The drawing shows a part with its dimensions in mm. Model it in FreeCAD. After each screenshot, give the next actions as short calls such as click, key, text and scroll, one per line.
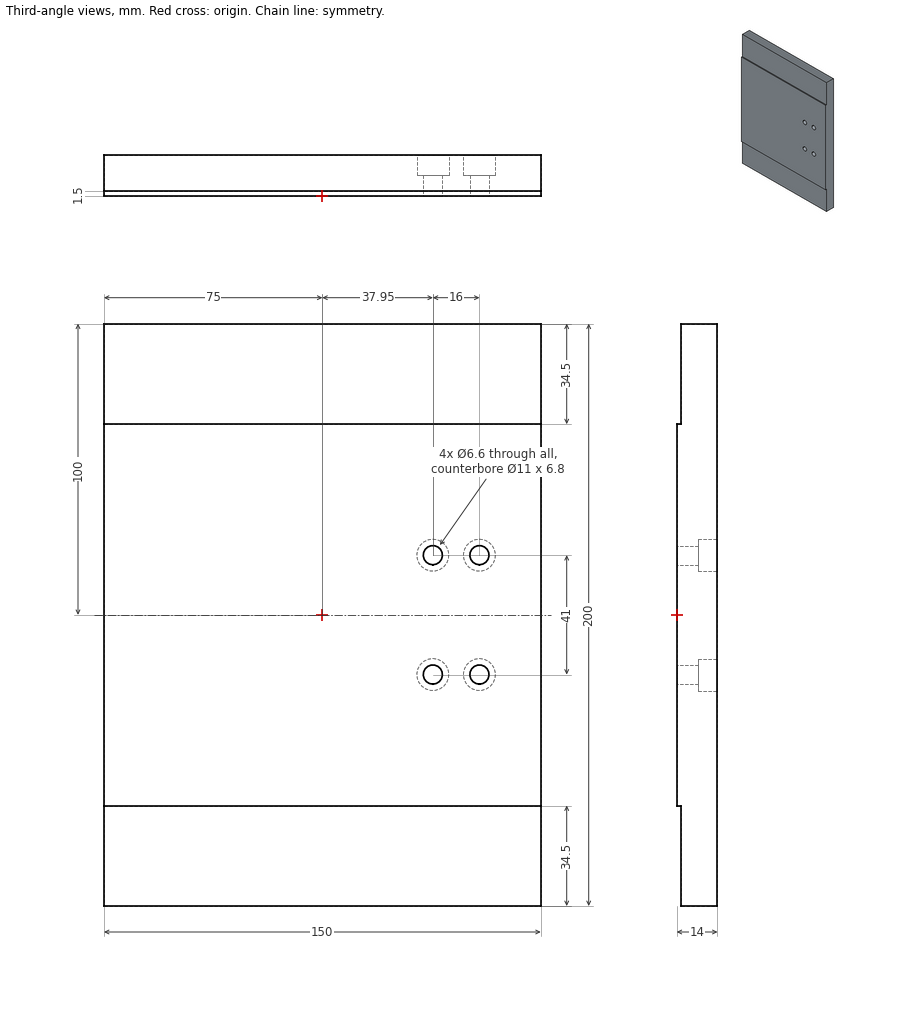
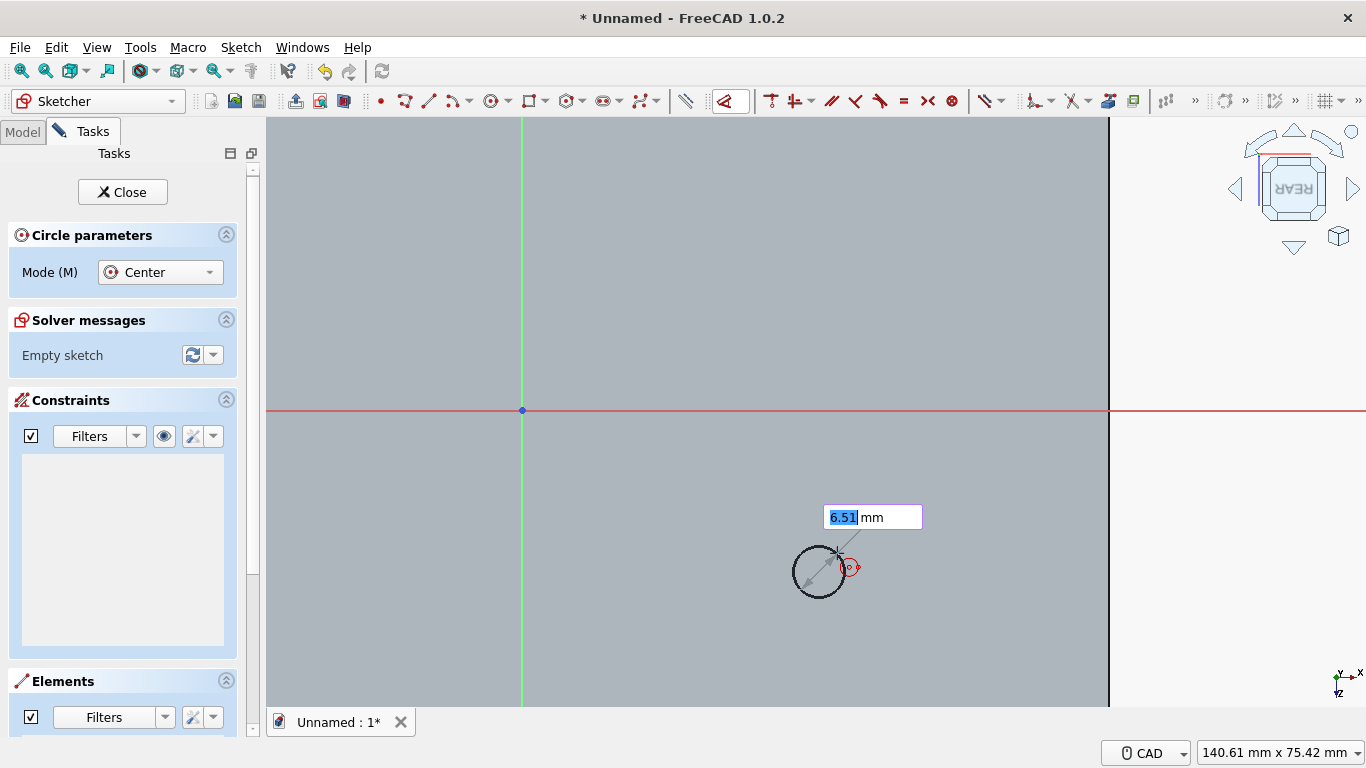
text(6.6)
key(Return)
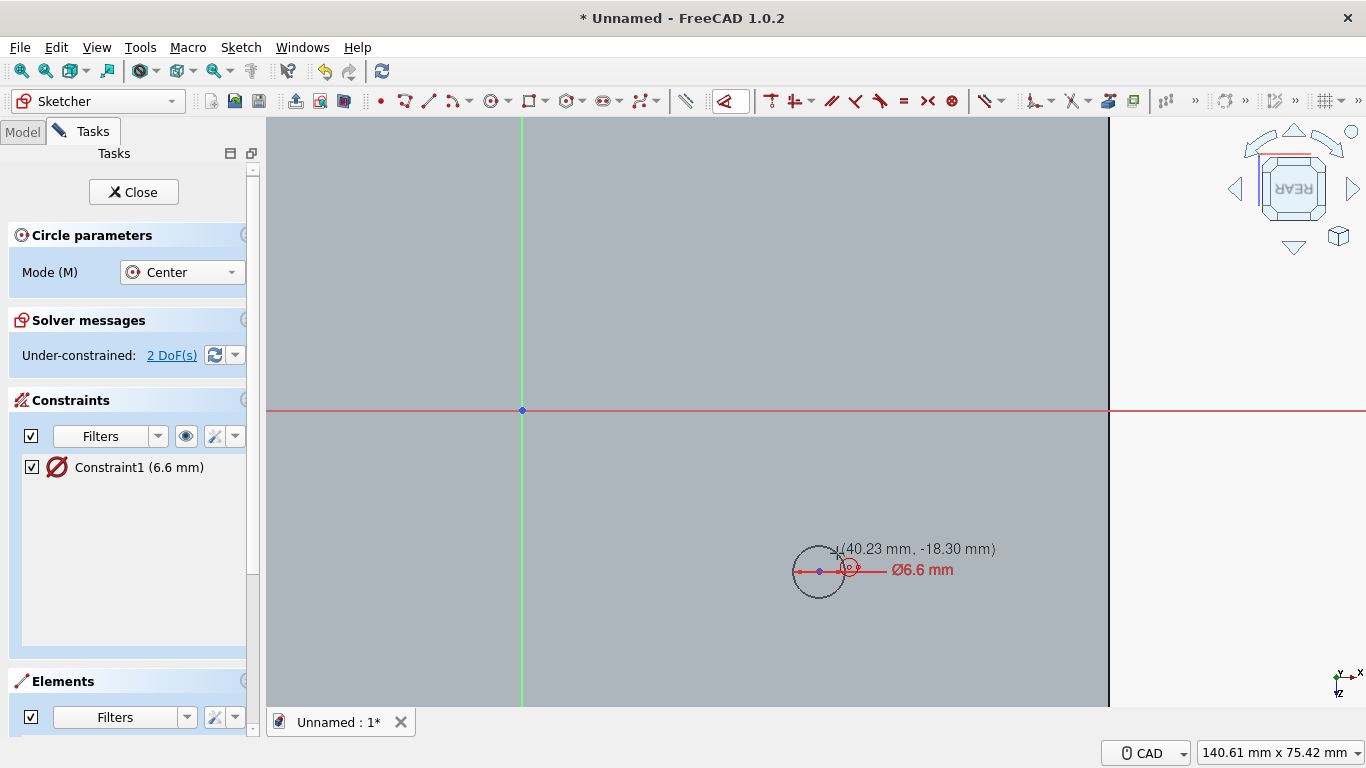
click(819, 250)
move(837, 232)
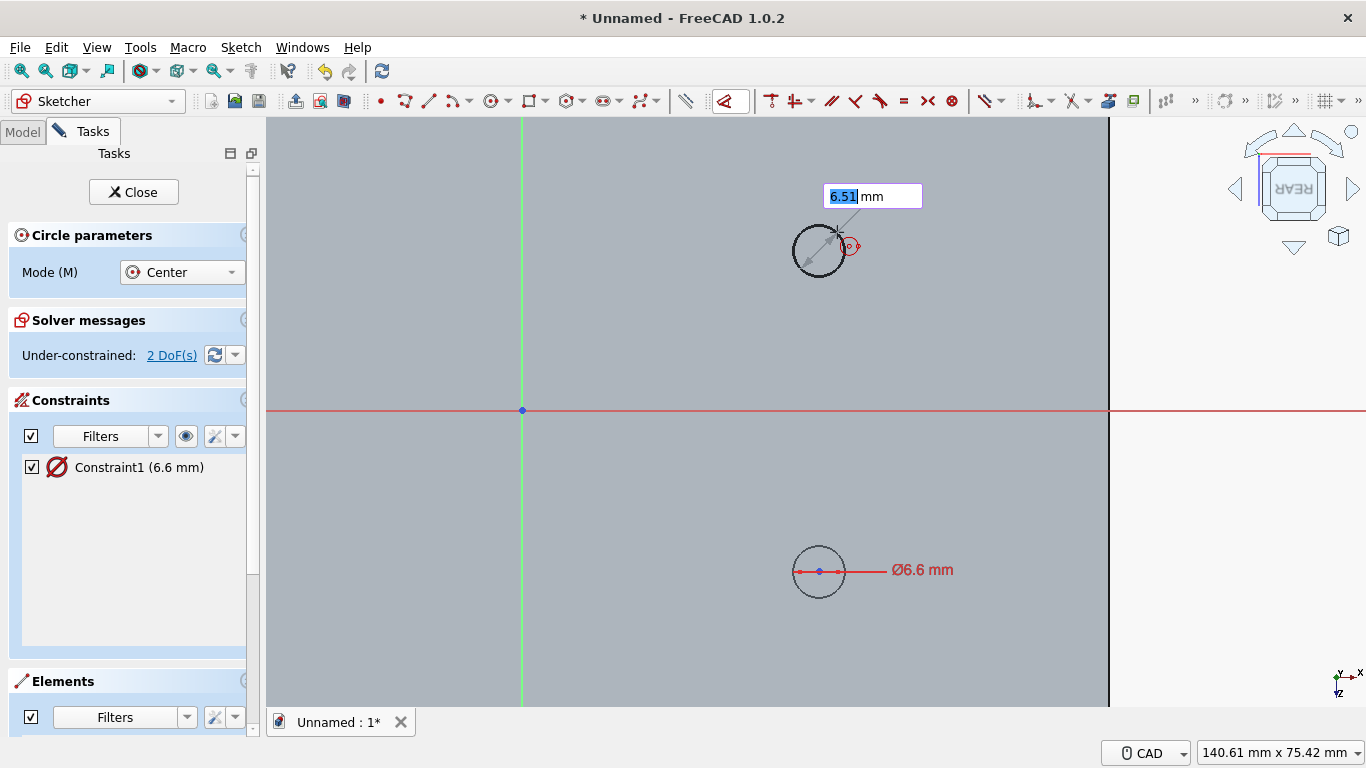
text(6.6)
key(Return)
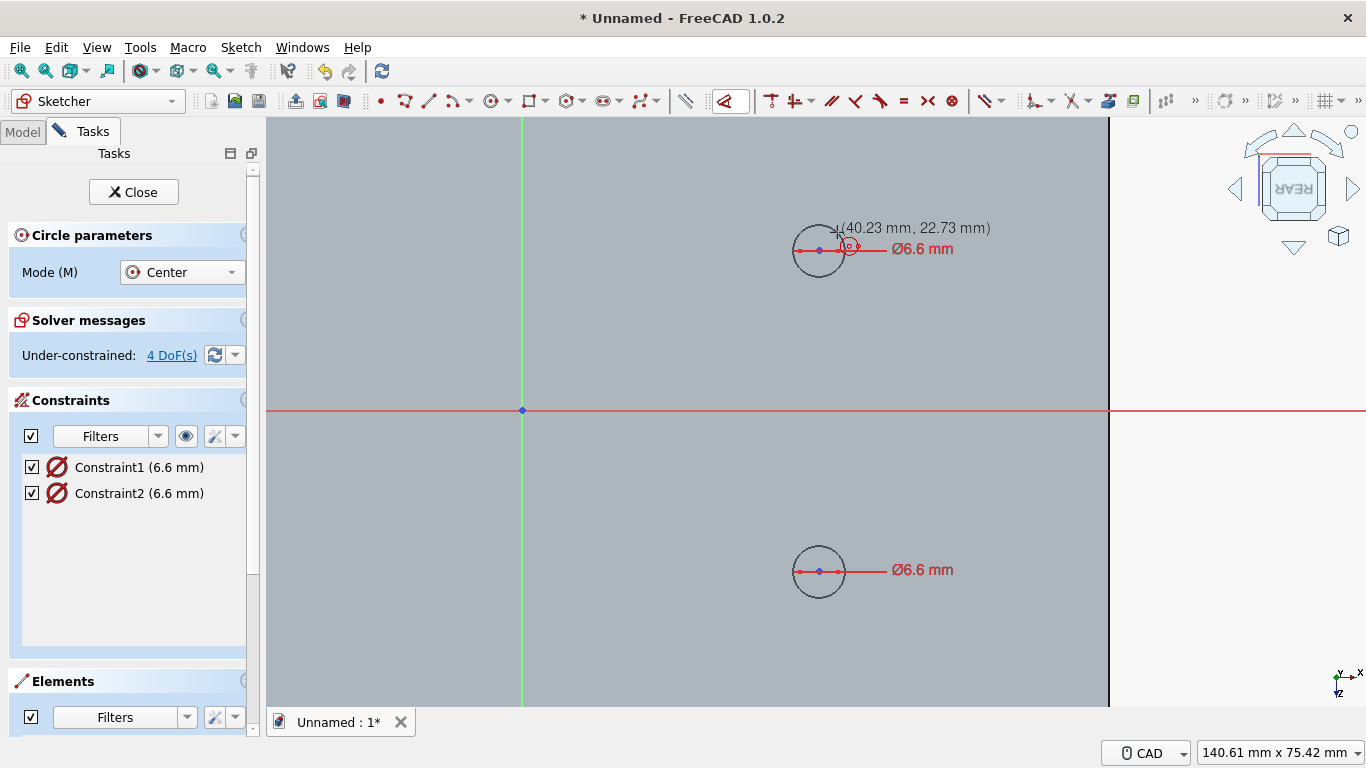
click(944, 571)
move(963, 553)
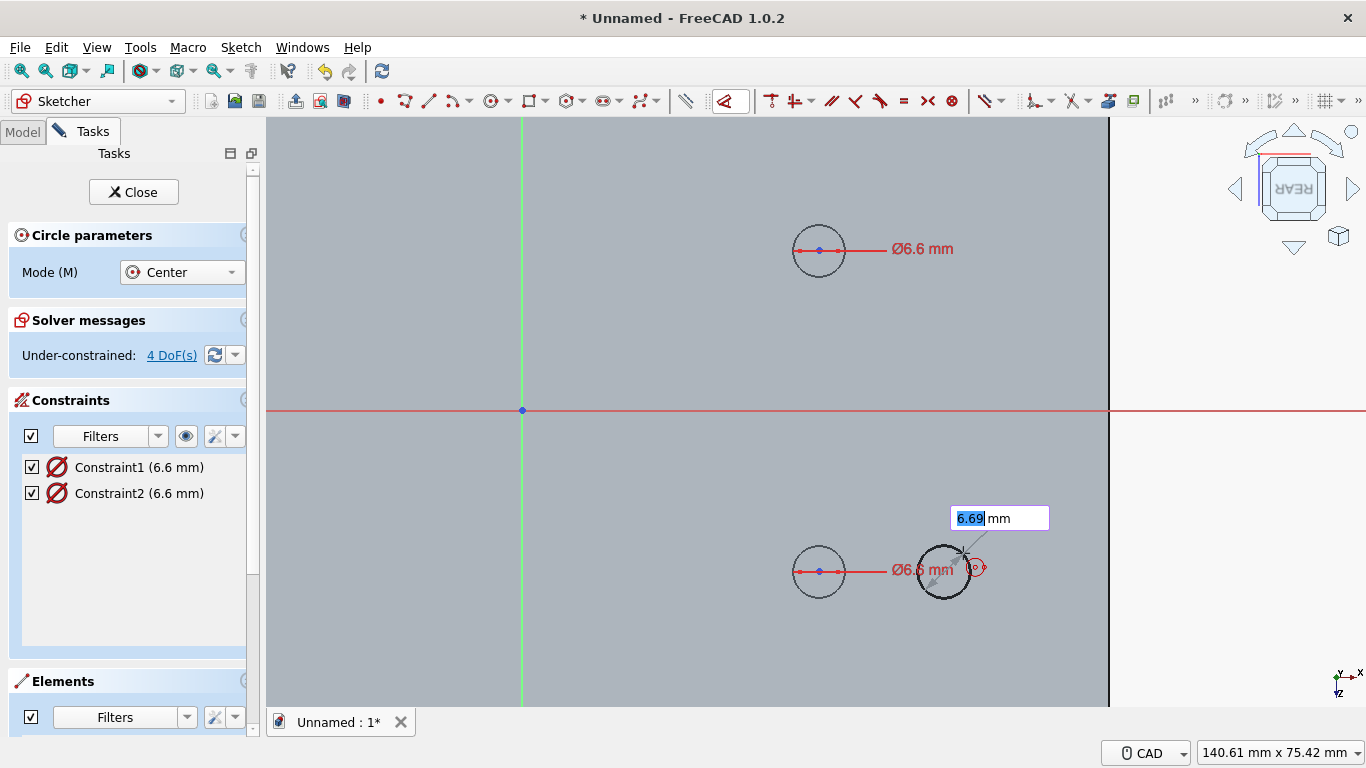
text(6.6)
key(Return)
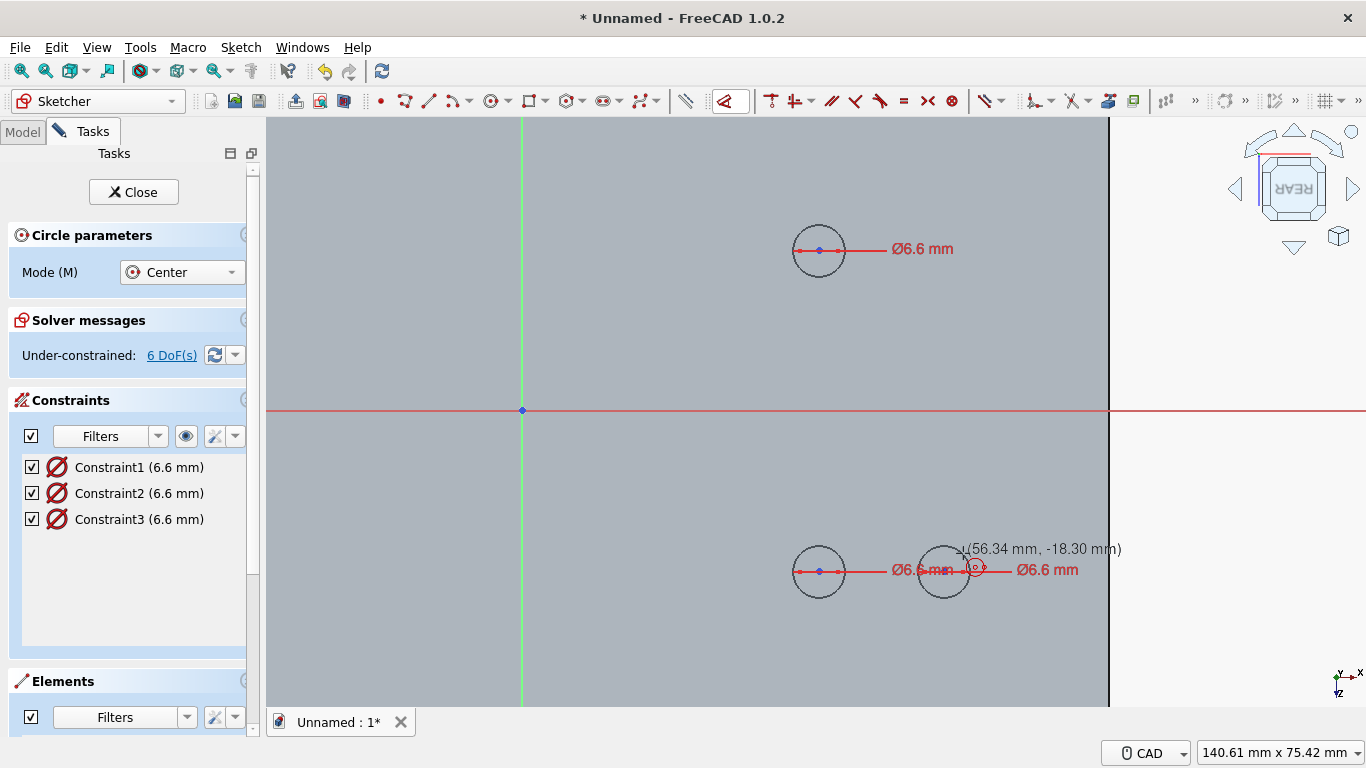
click(944, 250)
move(963, 232)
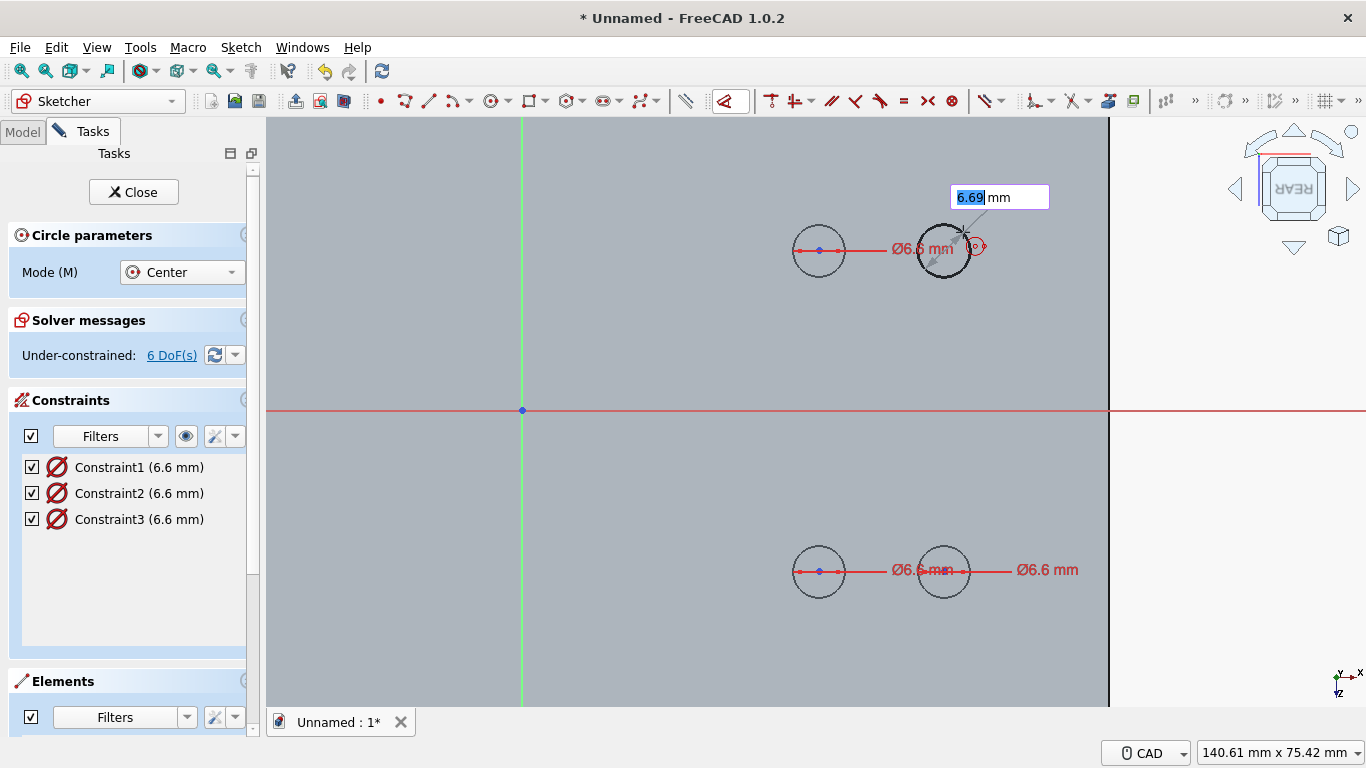
text(6.6)
key(Return)
key(Escape)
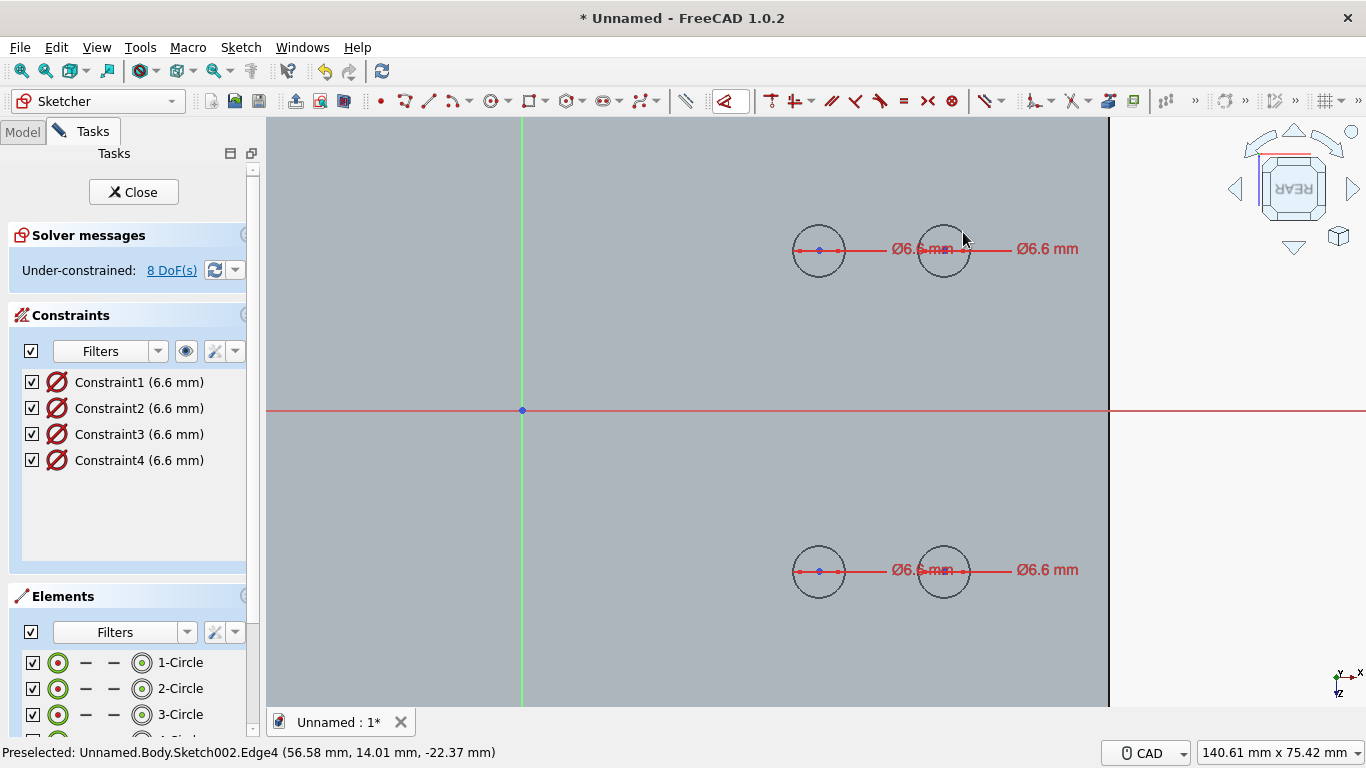
click(819, 572)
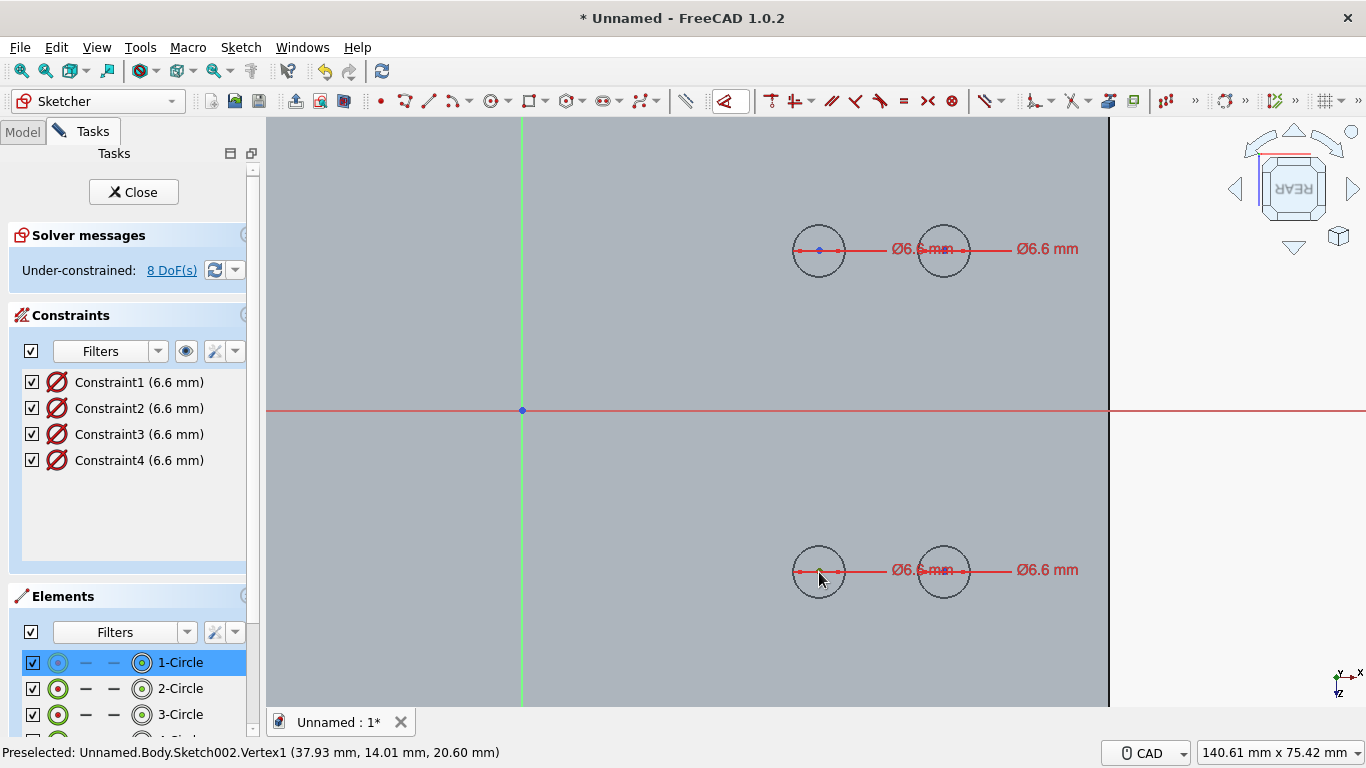
click(819, 251)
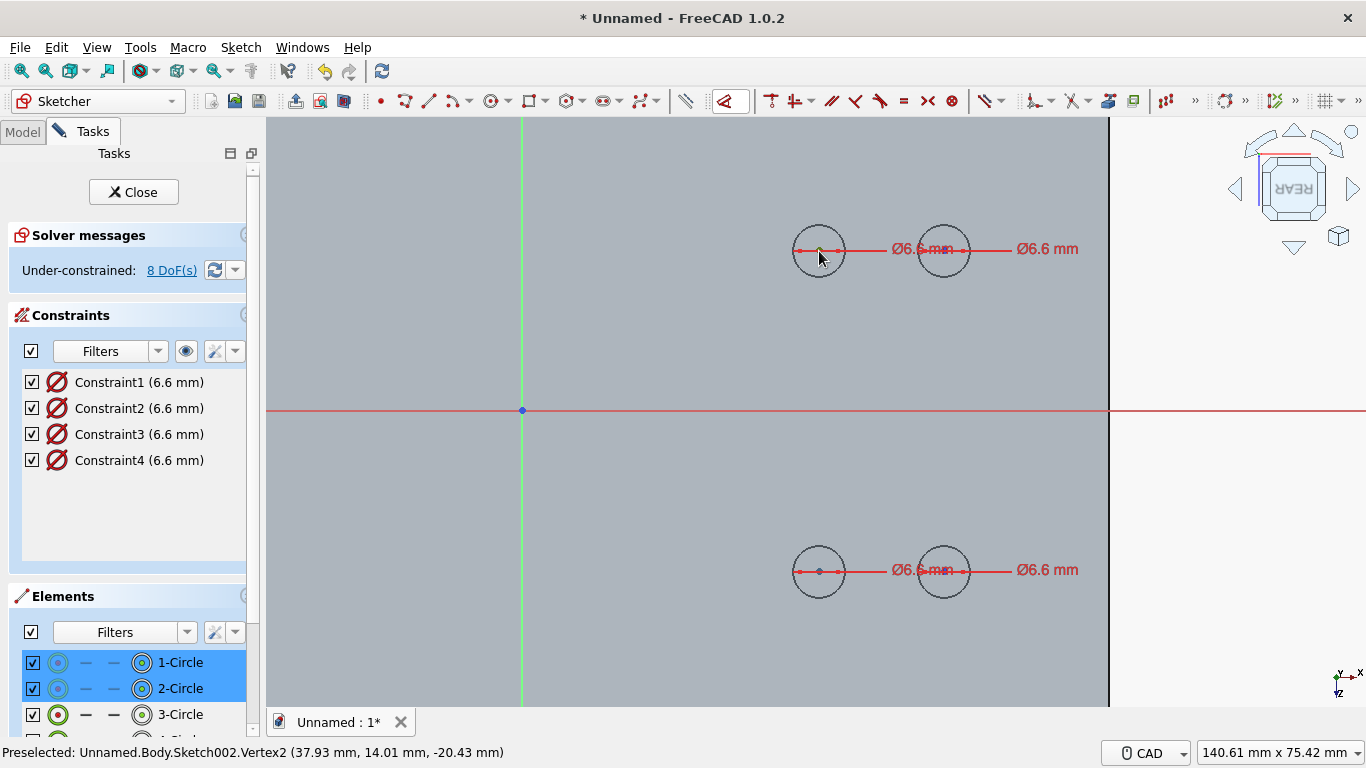
click(359, 411)